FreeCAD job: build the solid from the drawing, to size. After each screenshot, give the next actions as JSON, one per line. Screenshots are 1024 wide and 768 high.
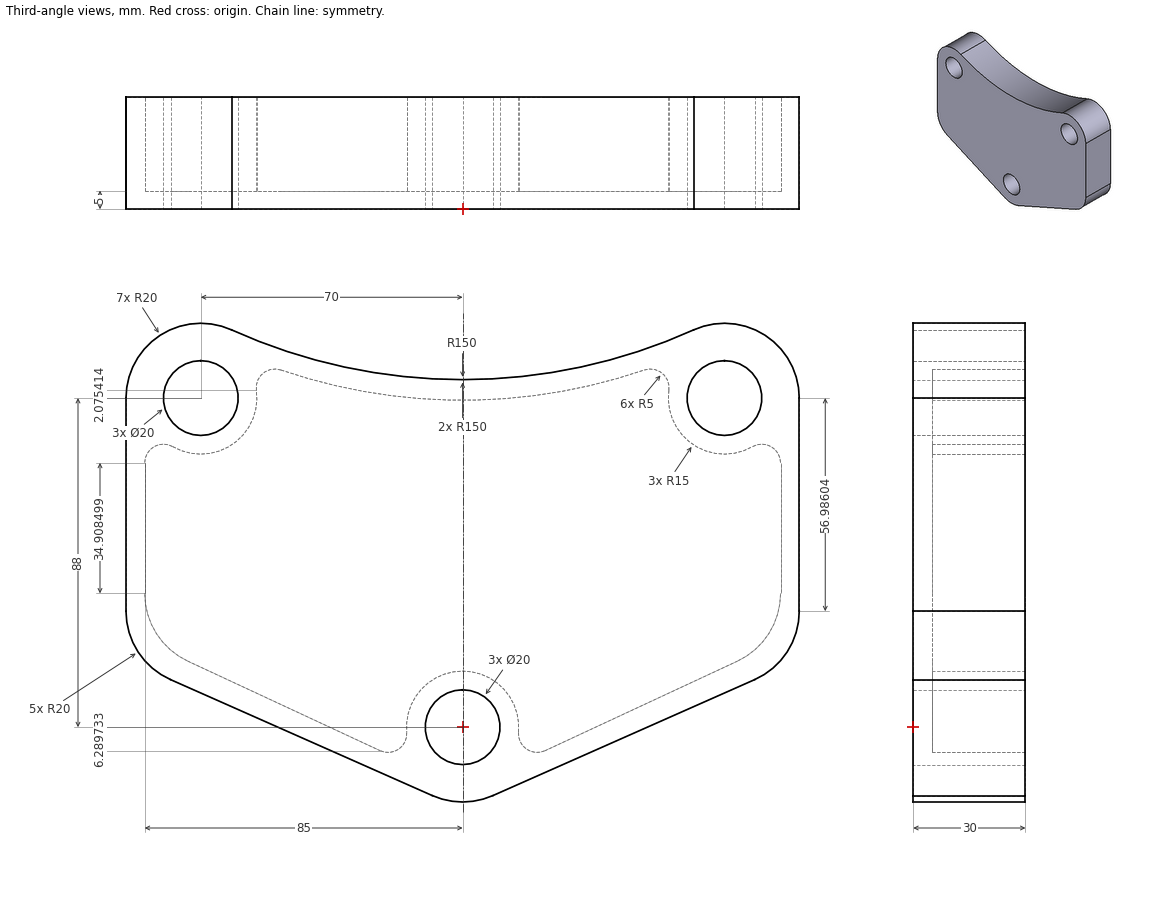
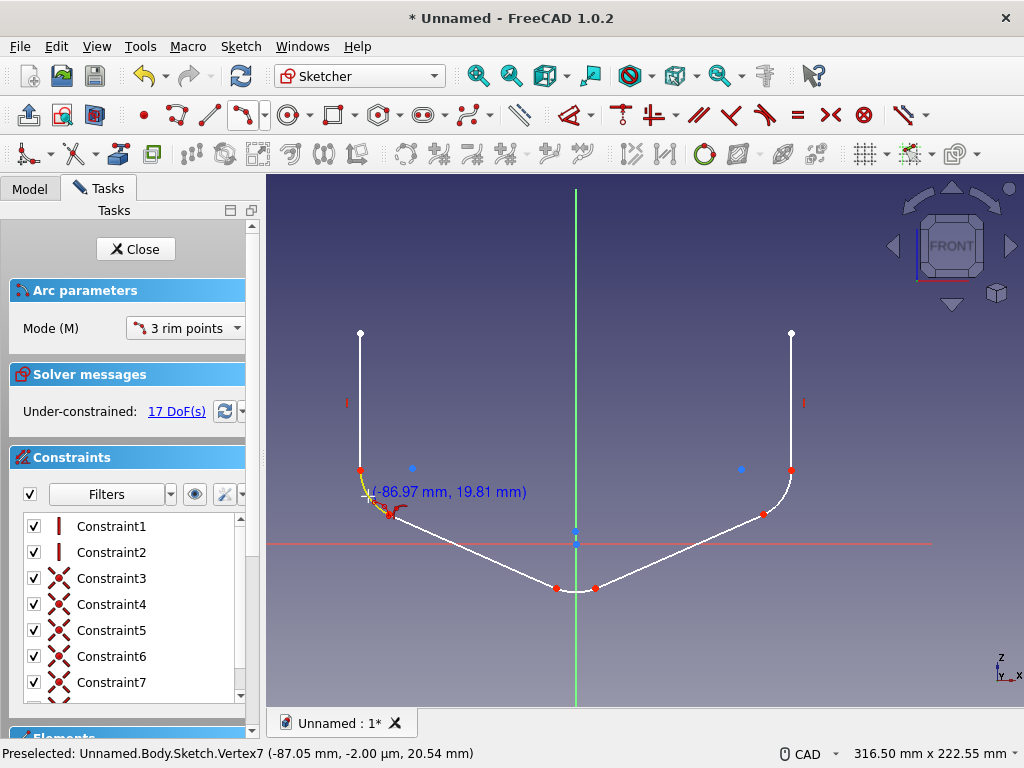
{"action": "left_click", "coordinate": [360, 334]}
{"action": "left_click", "coordinate": [428, 290]}
{"action": "left_click", "coordinate": [383, 293]}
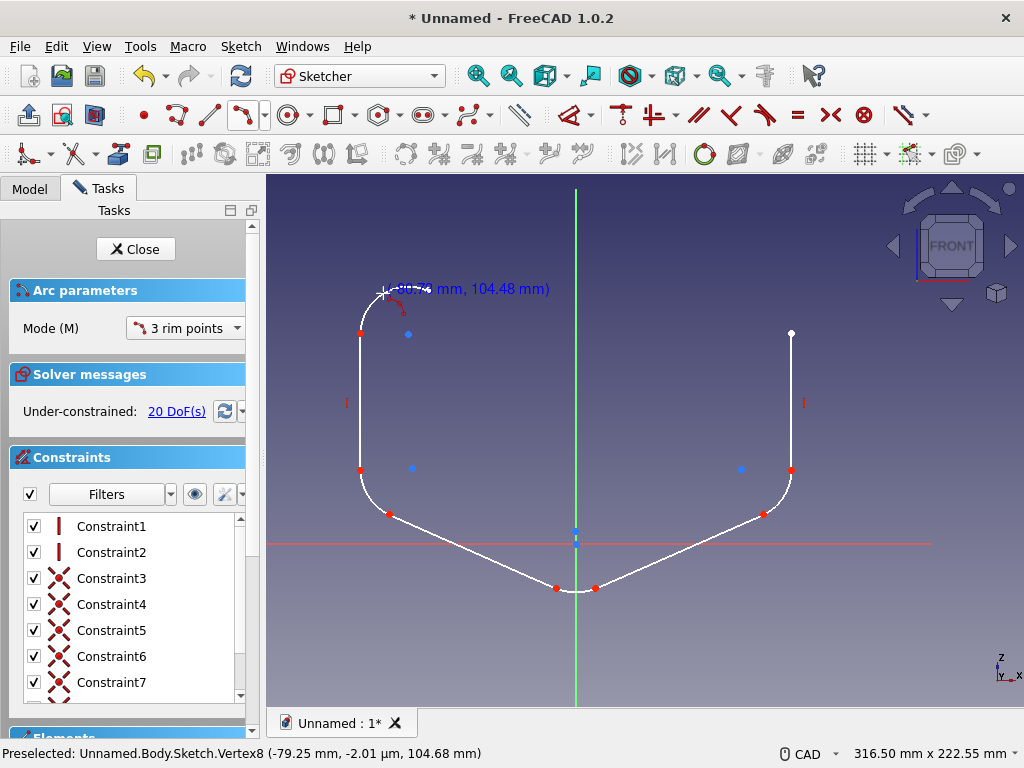
{"action": "left_click", "coordinate": [428, 291]}
{"action": "left_click", "coordinate": [724, 290]}
{"action": "left_click", "coordinate": [546, 320]}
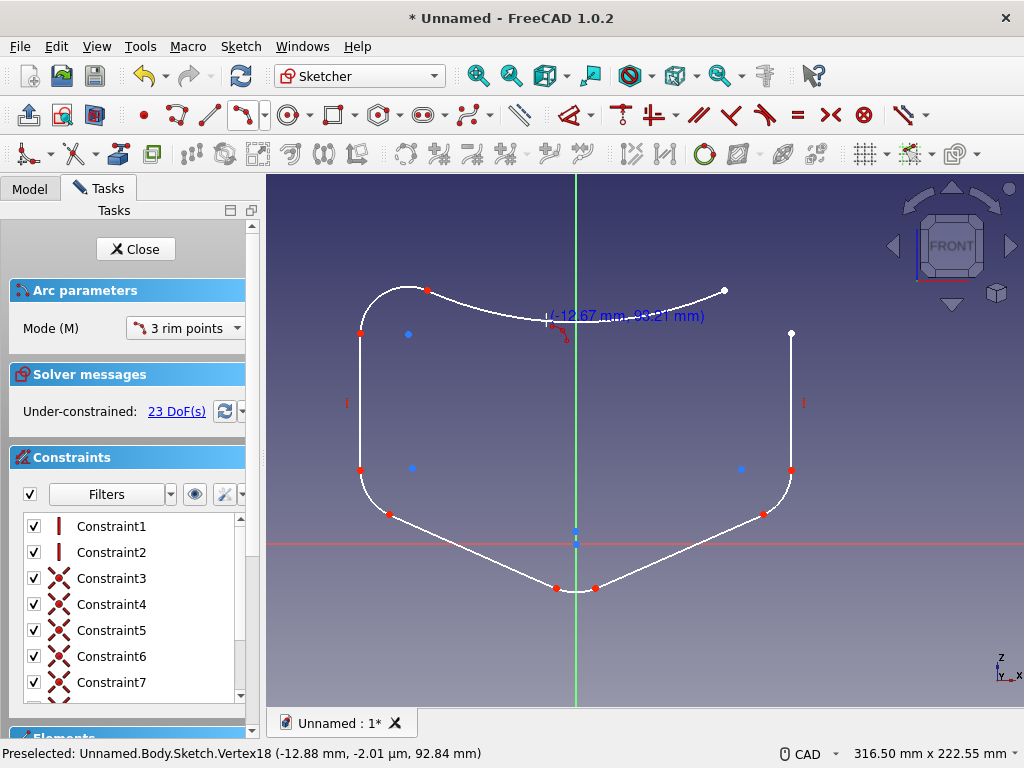
{"action": "left_click", "coordinate": [724, 291]}
{"action": "left_click", "coordinate": [791, 334]}
{"action": "left_click", "coordinate": [770, 293]}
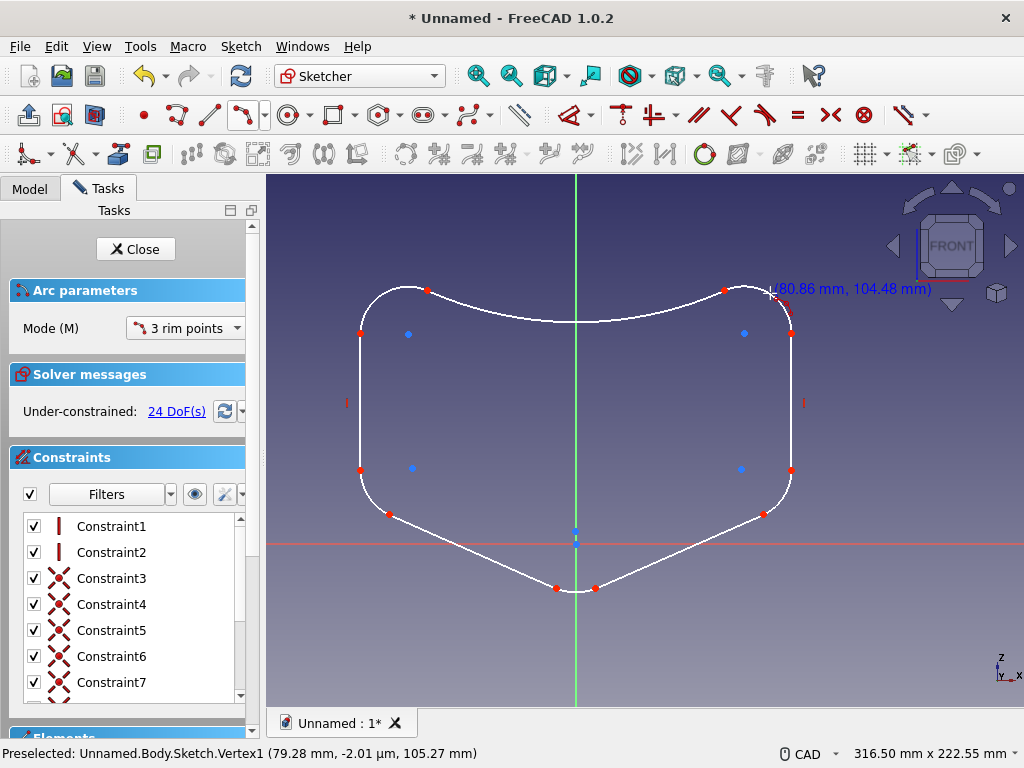
{"action": "left_click", "coordinate": [210, 116]}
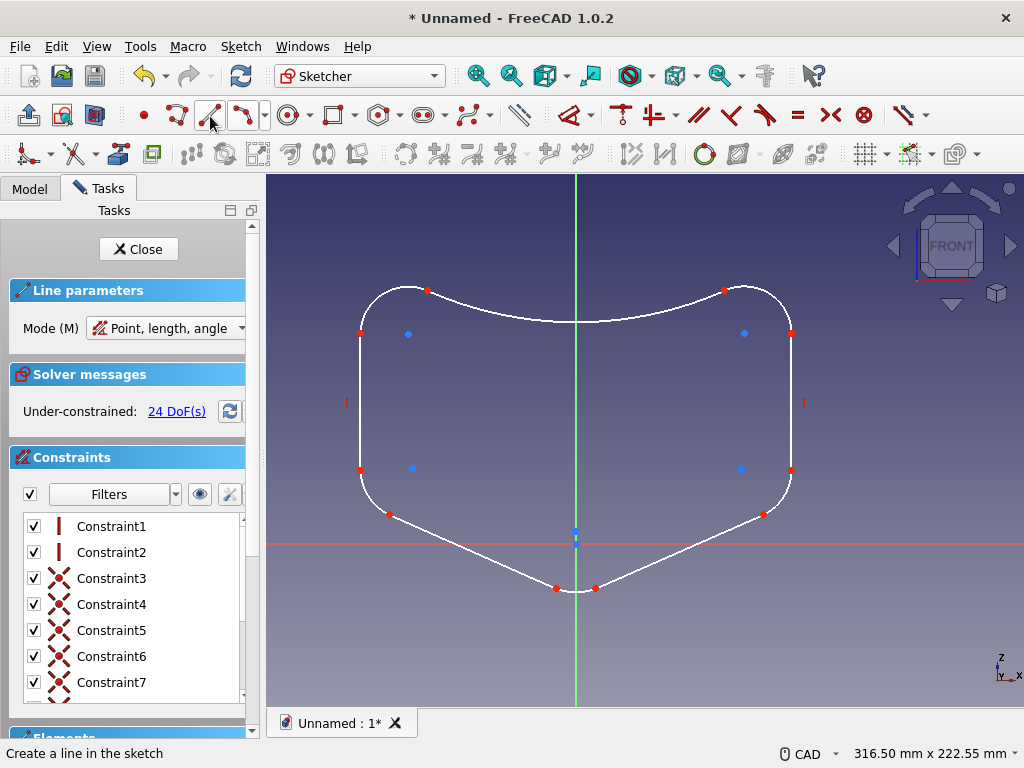
{"action": "scroll", "coordinate": [373, 375], "scroll_direction": "up", "scroll_amount": 2}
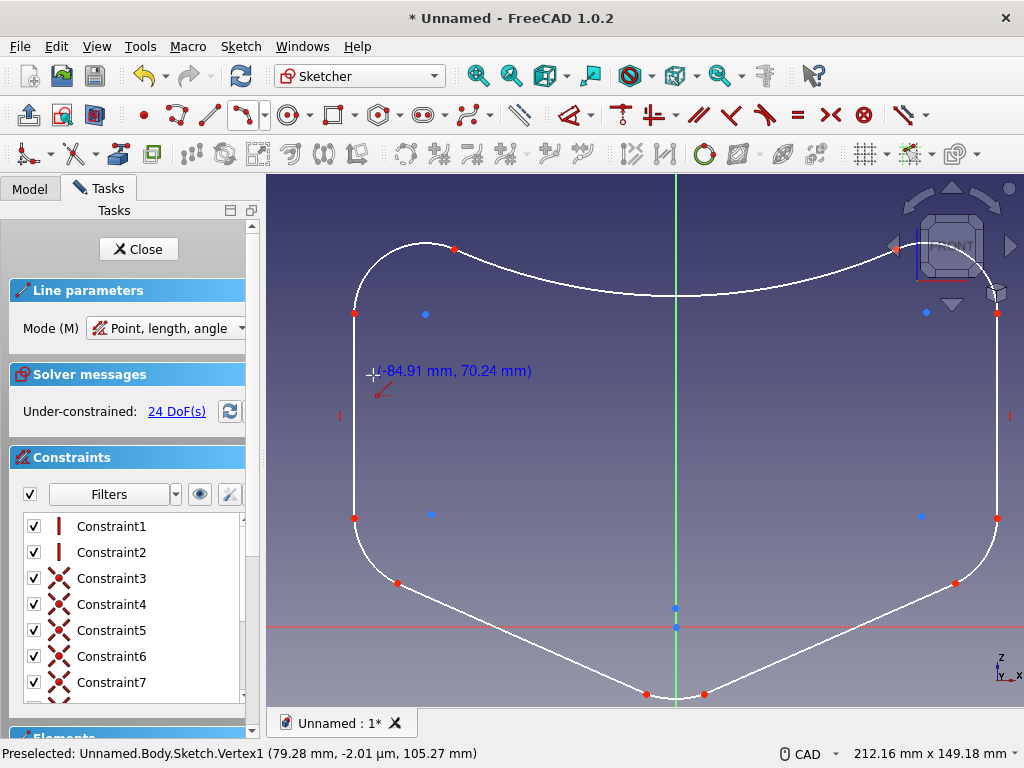
{"action": "left_click", "coordinate": [373, 375]}
{"action": "left_click", "coordinate": [373, 499]}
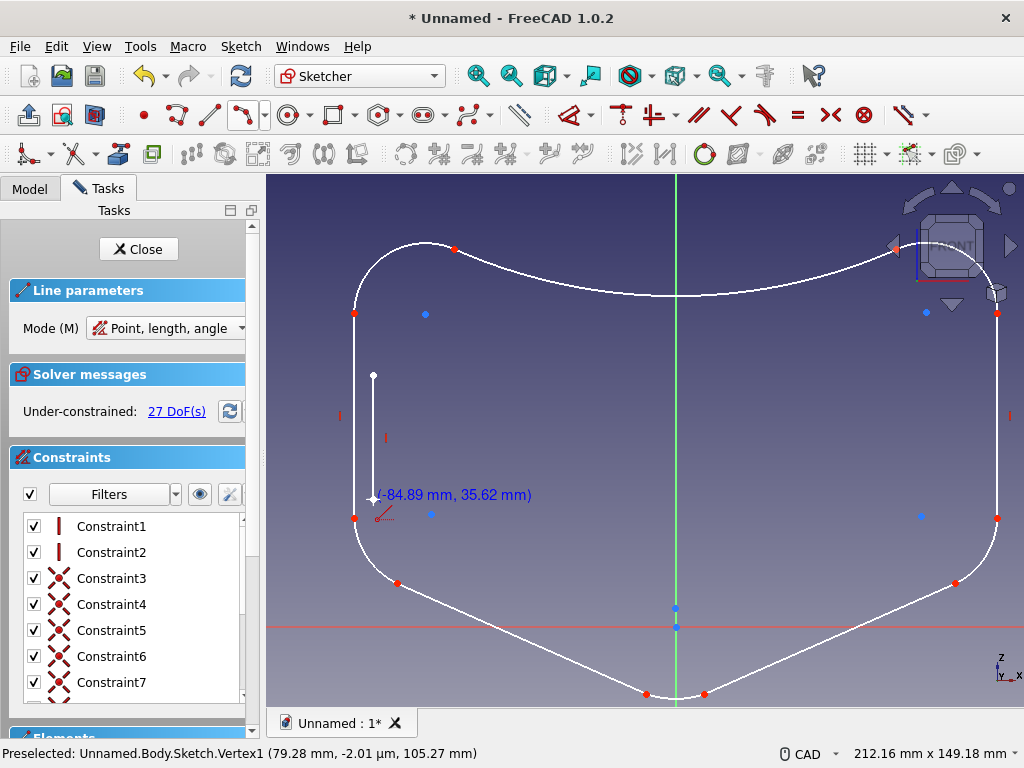
{"action": "left_click", "coordinate": [414, 564]}
{"action": "left_click", "coordinate": [598, 650]}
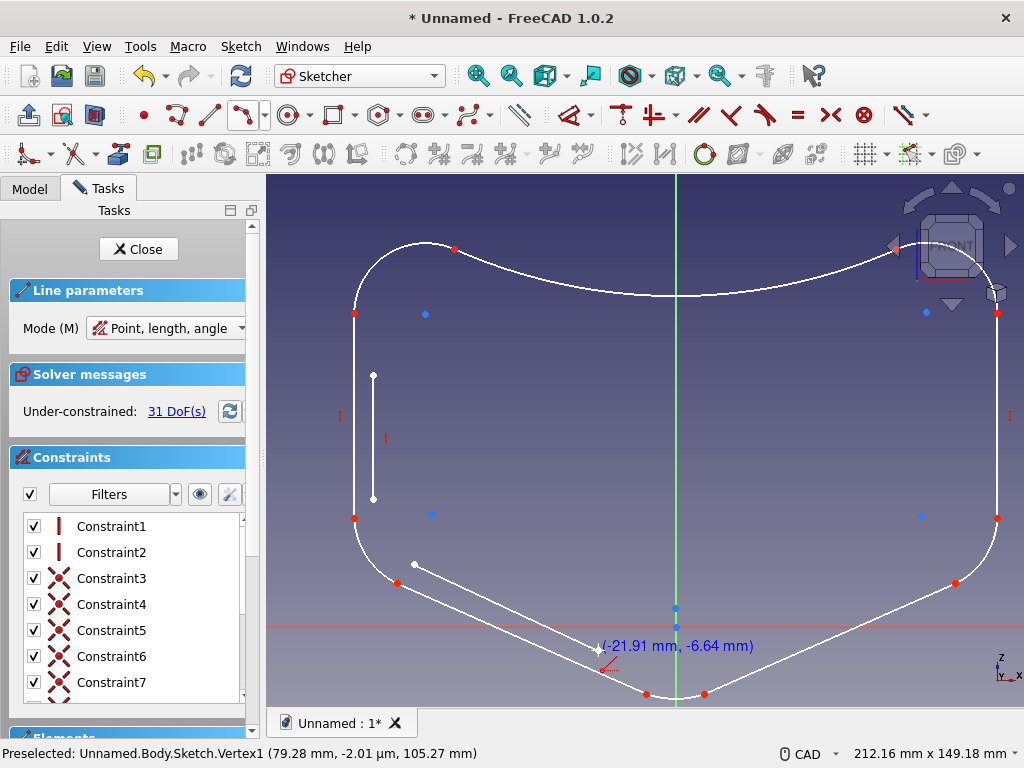
{"action": "left_click", "coordinate": [755, 650]}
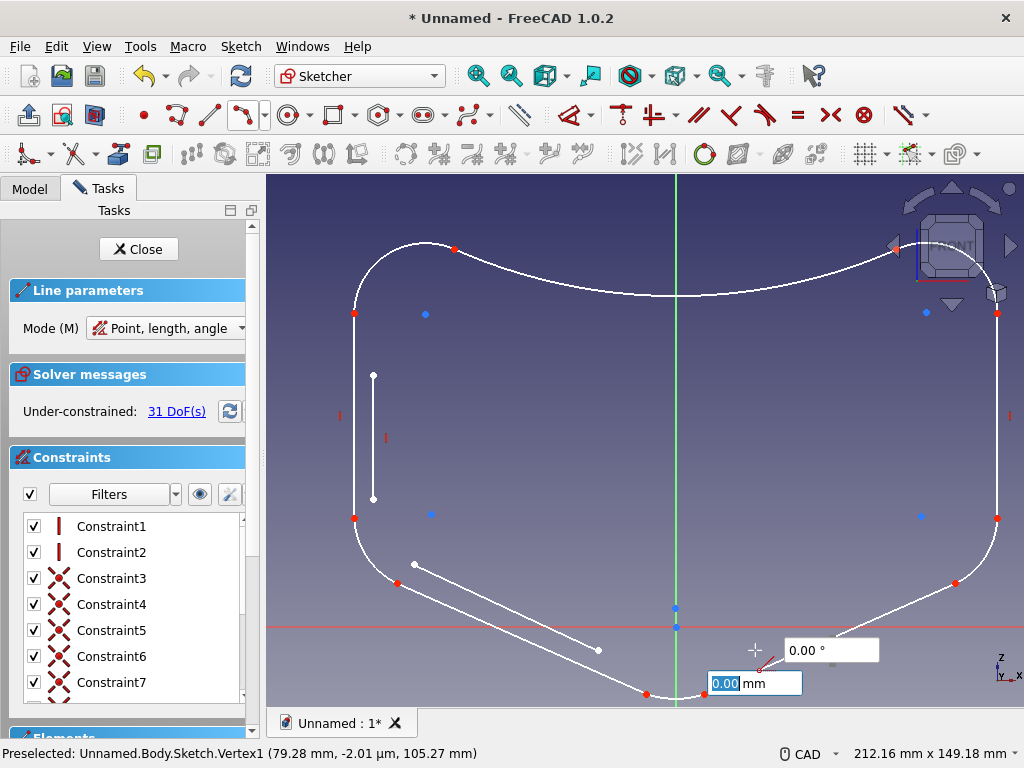
{"action": "scroll", "coordinate": [374, 374], "scroll_direction": "down", "scroll_amount": 2}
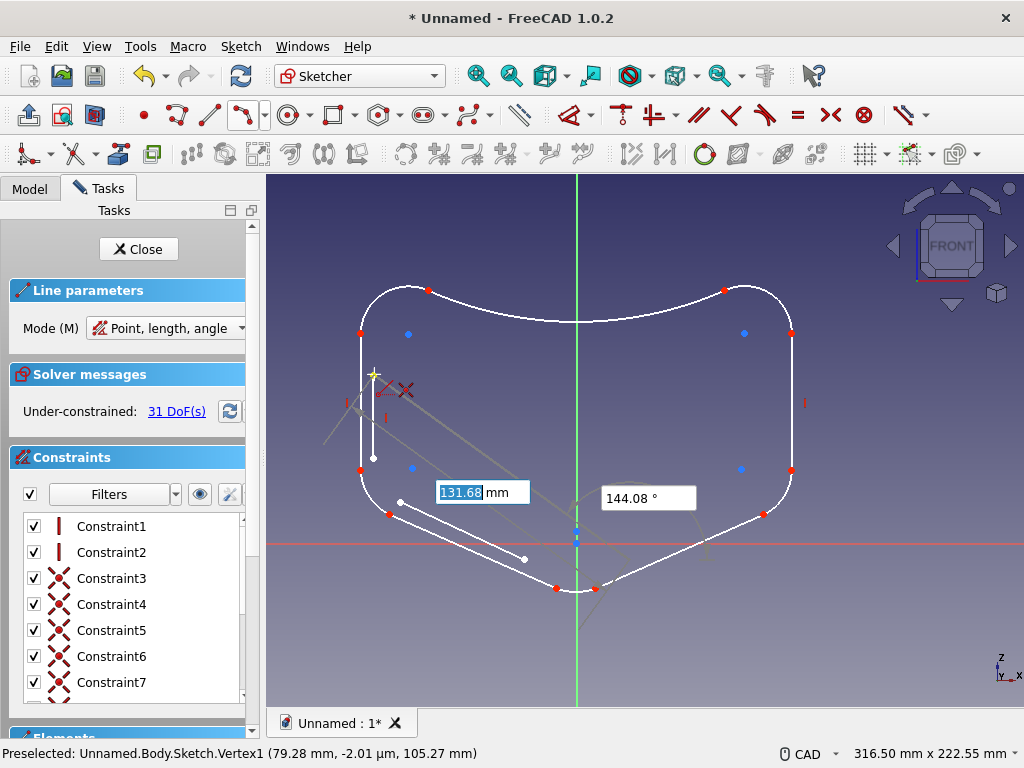
{"action": "left_click", "coordinate": [753, 502]}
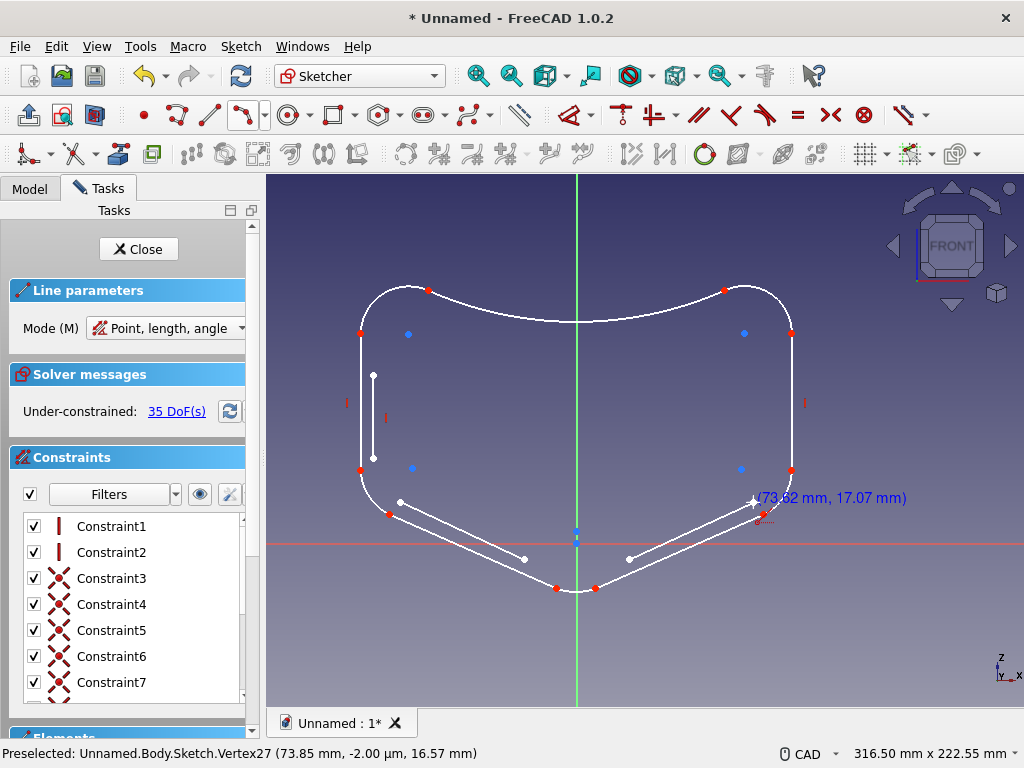
{"action": "scroll", "coordinate": [780, 458], "scroll_direction": "up", "scroll_amount": 2}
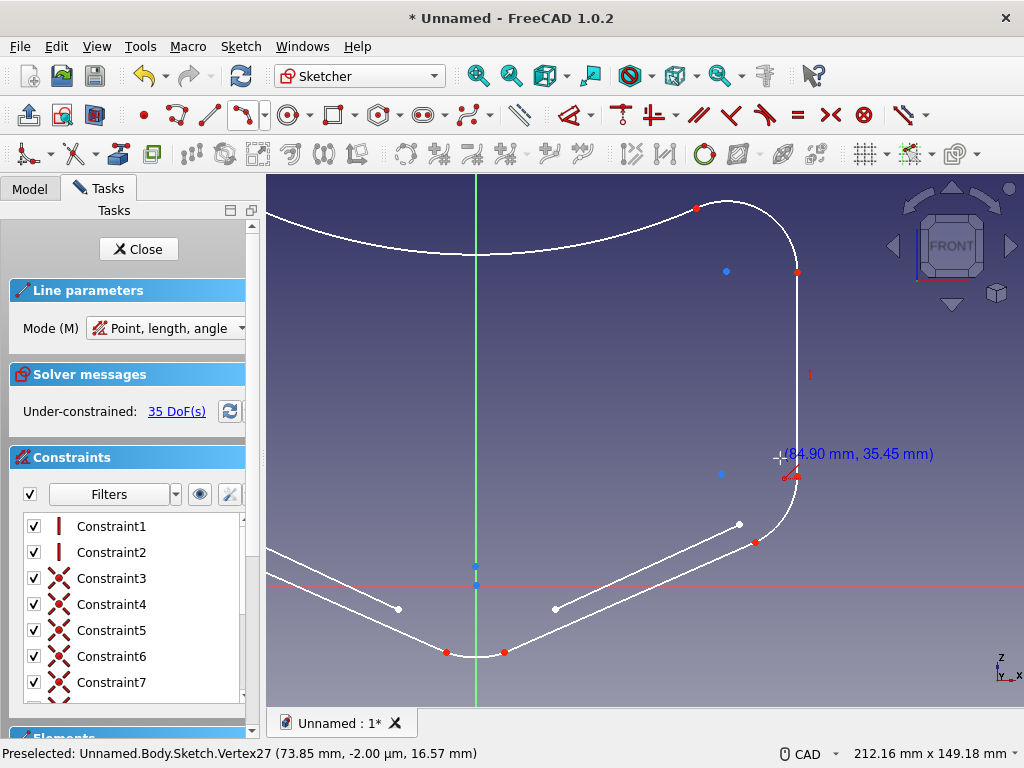
{"action": "left_click", "coordinate": [780, 458]}
{"action": "left_click", "coordinate": [780, 333]}